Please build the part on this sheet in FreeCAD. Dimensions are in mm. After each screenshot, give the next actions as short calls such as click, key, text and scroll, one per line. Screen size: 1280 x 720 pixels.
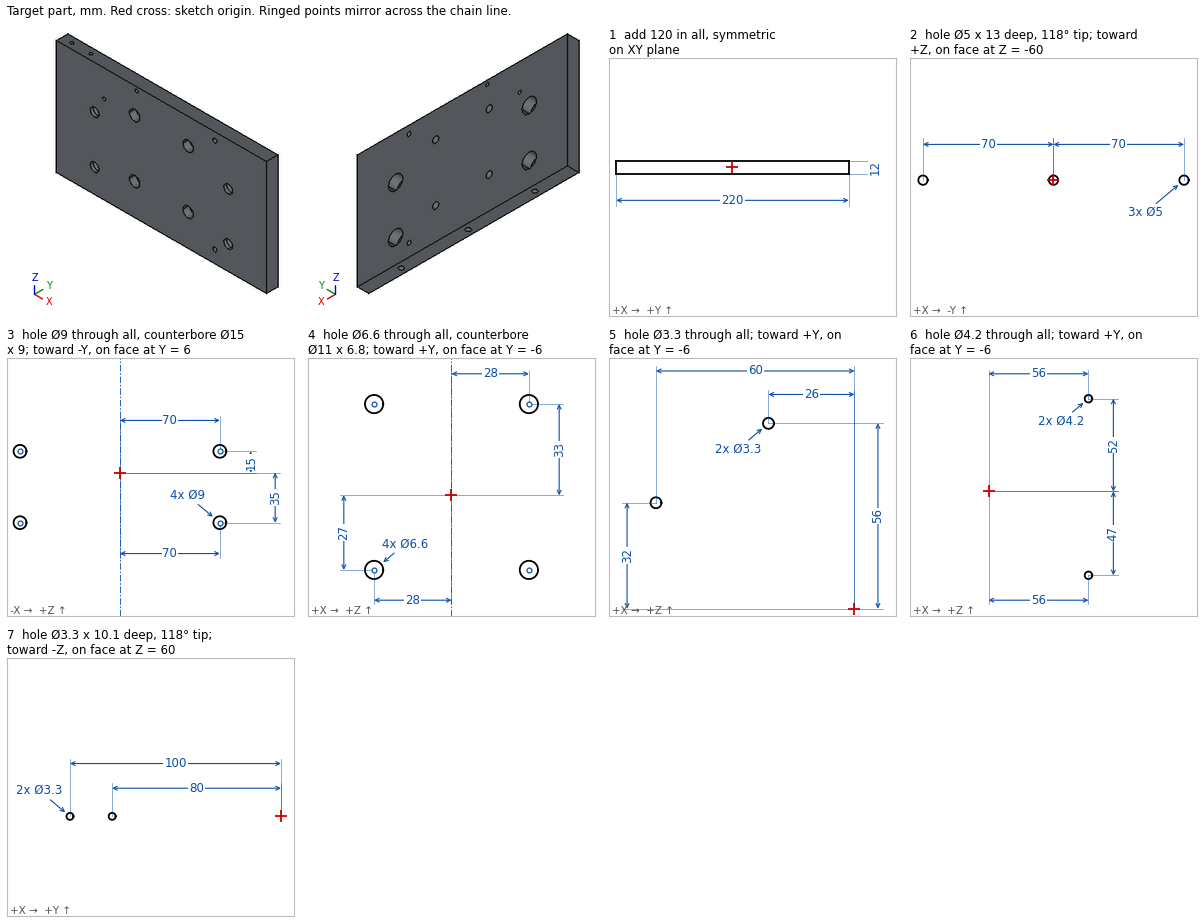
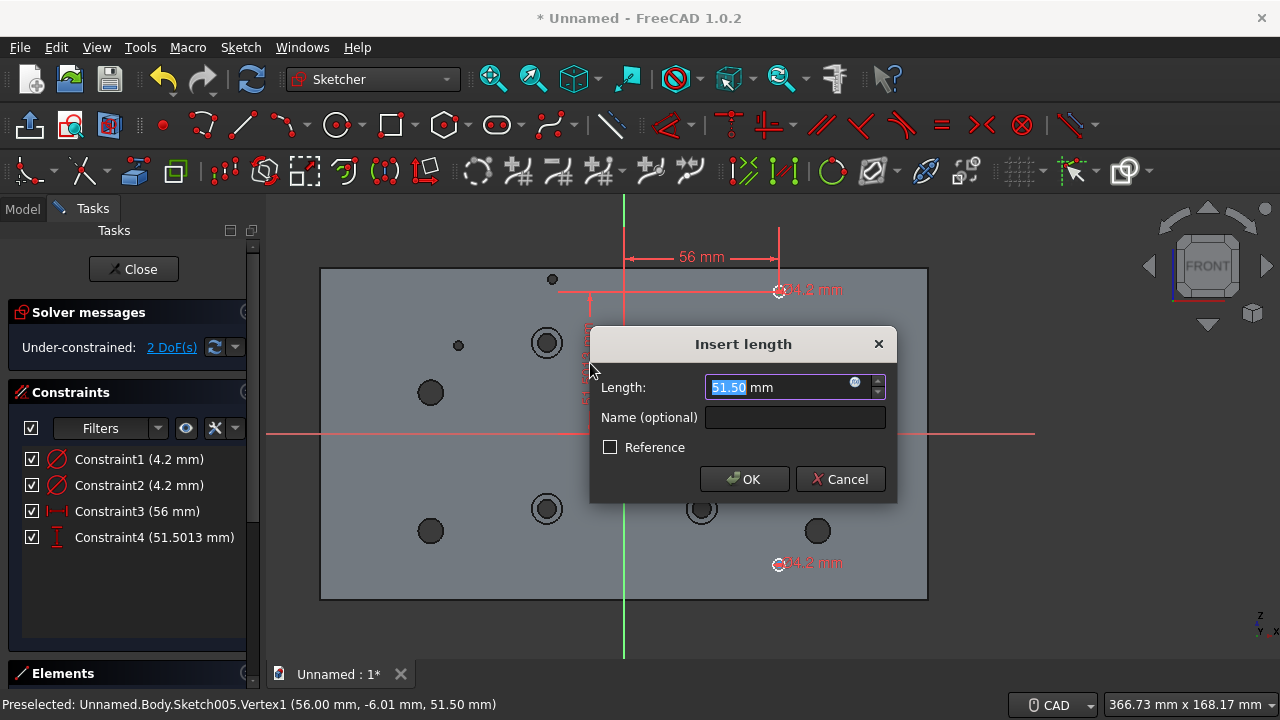
text(52)
key(Return)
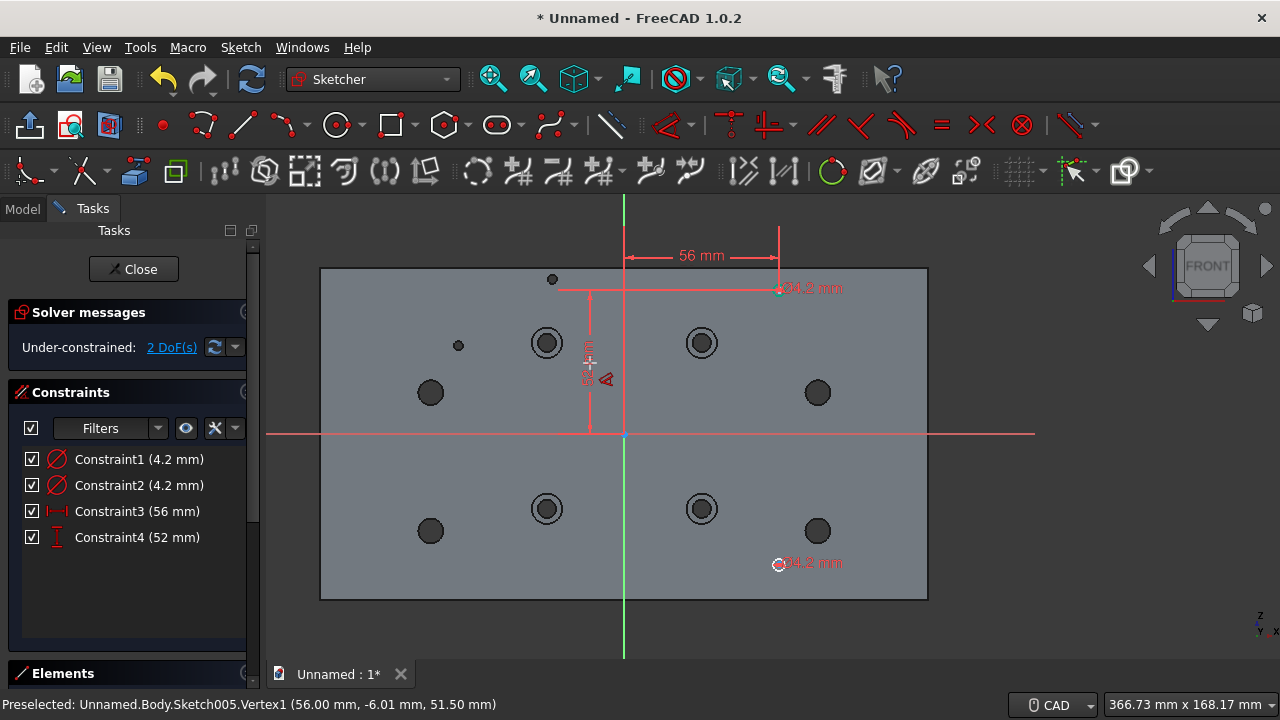
click(779, 565)
click(702, 599)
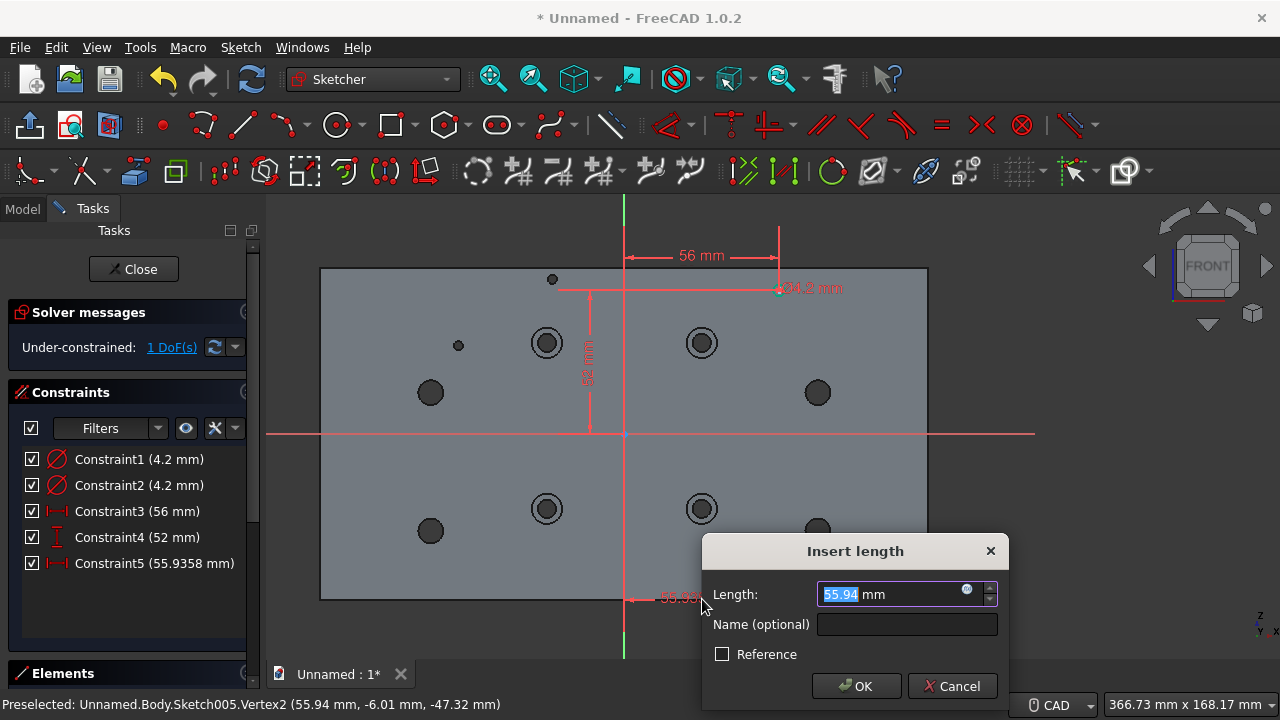
text(56)
key(Return)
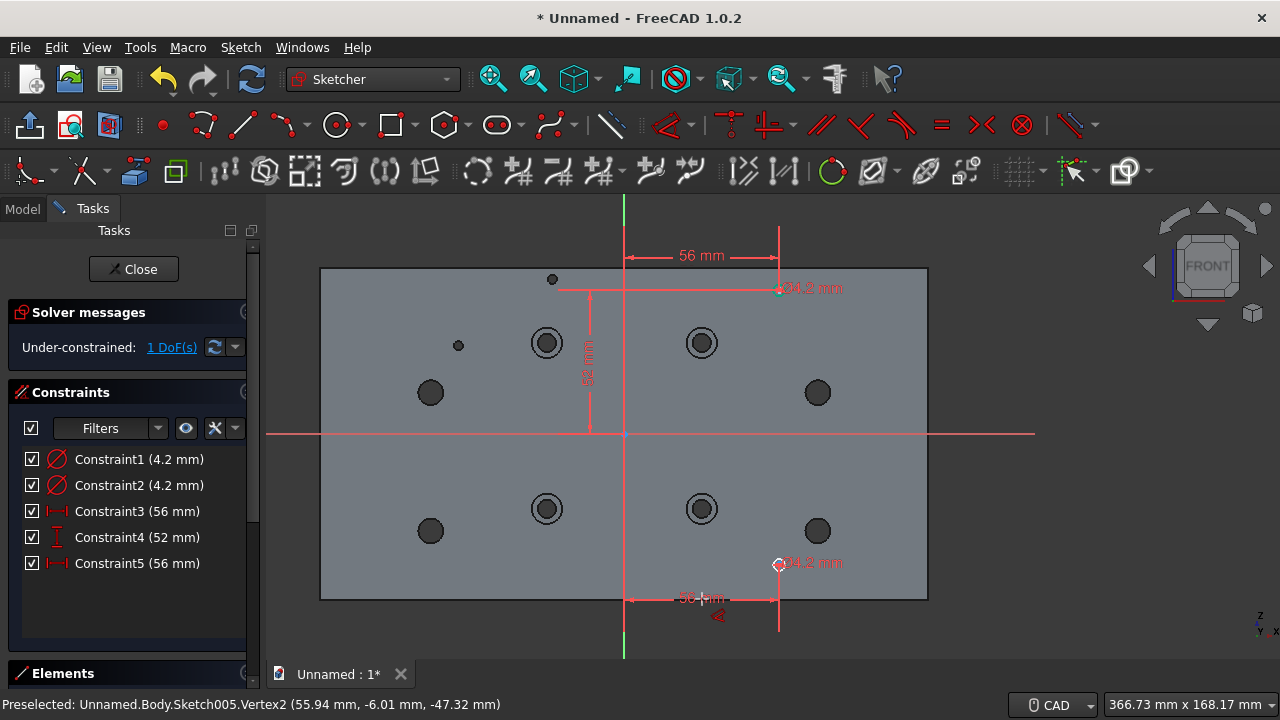
click(779, 565)
click(590, 500)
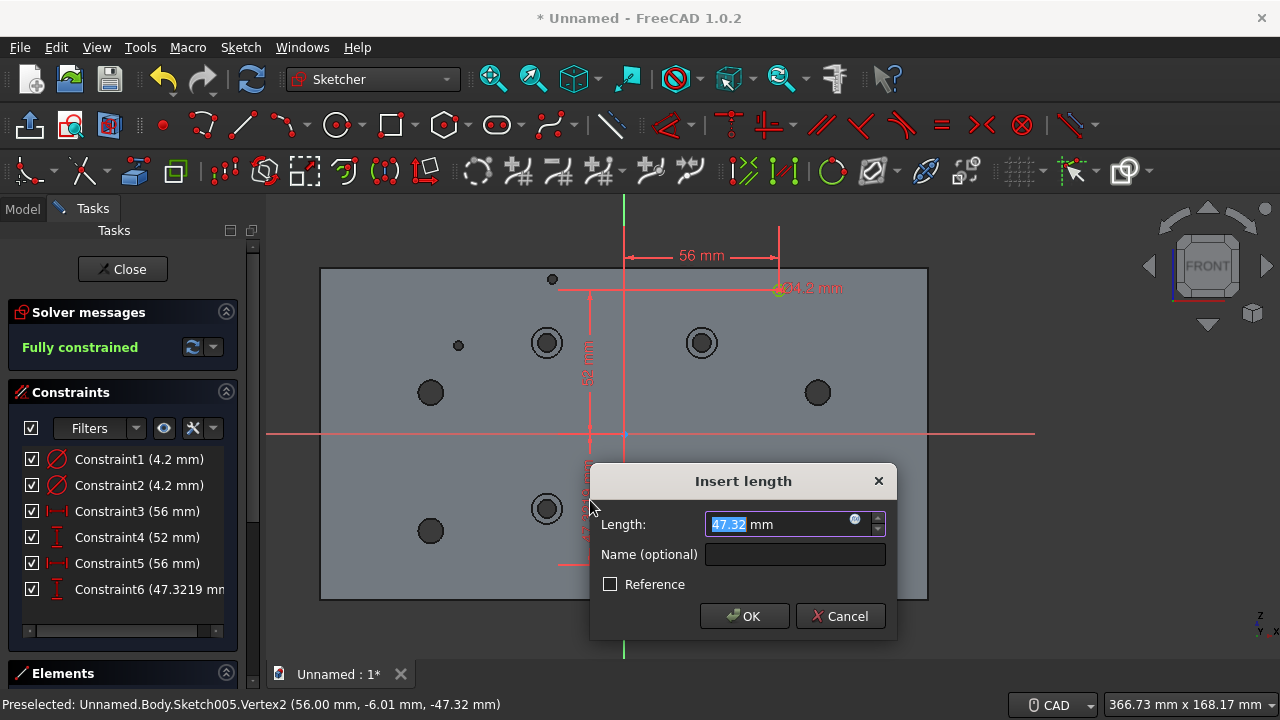
text(47)
key(Return)
key(Escape)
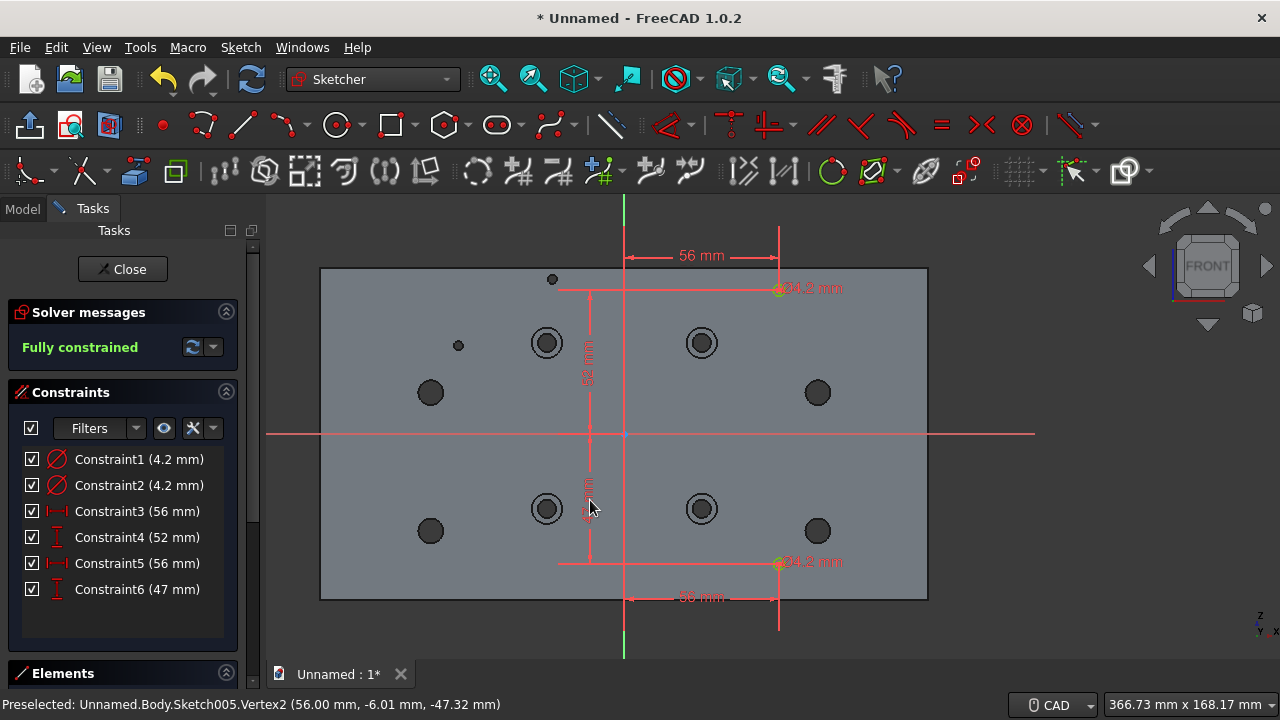
click(123, 269)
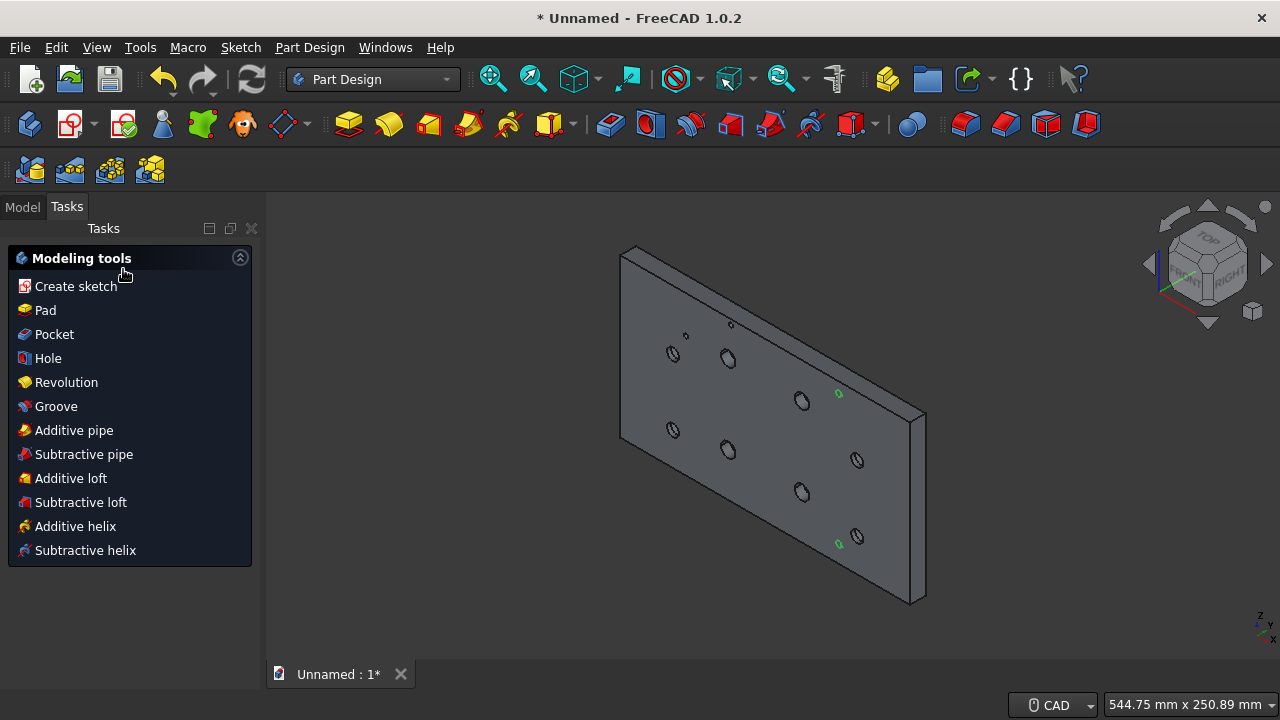
click(652, 124)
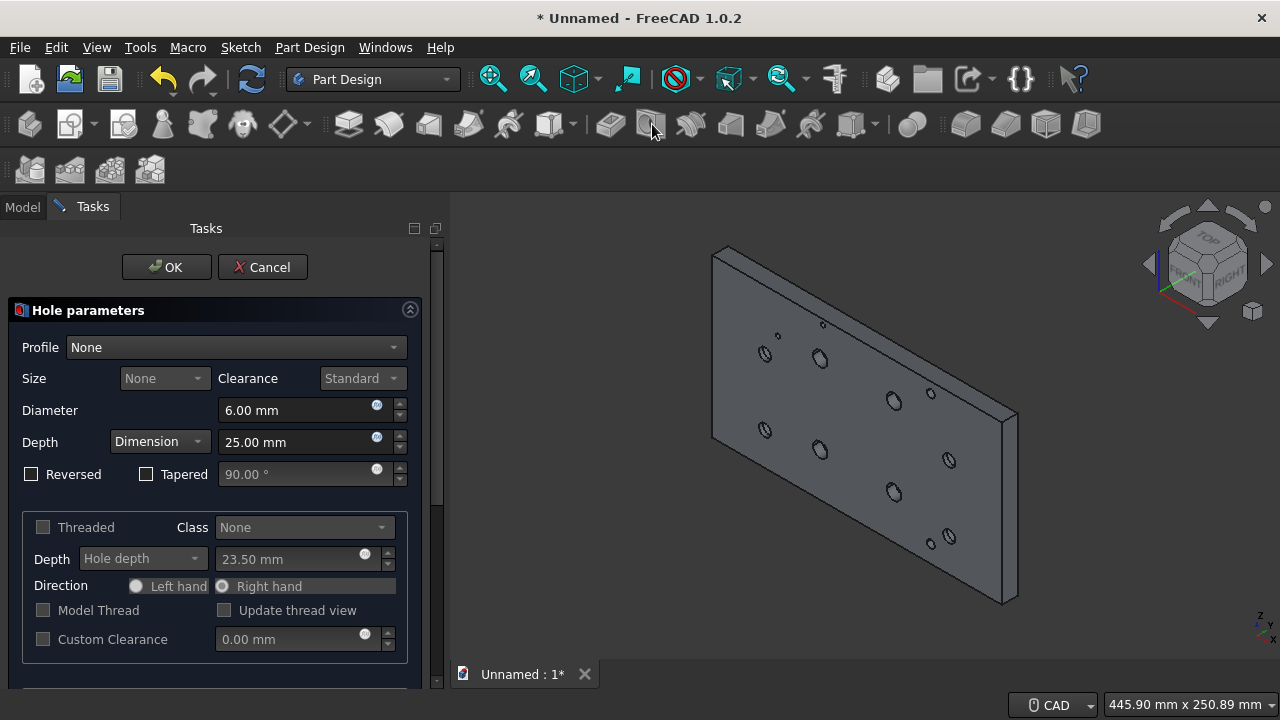
triple_click(305, 410)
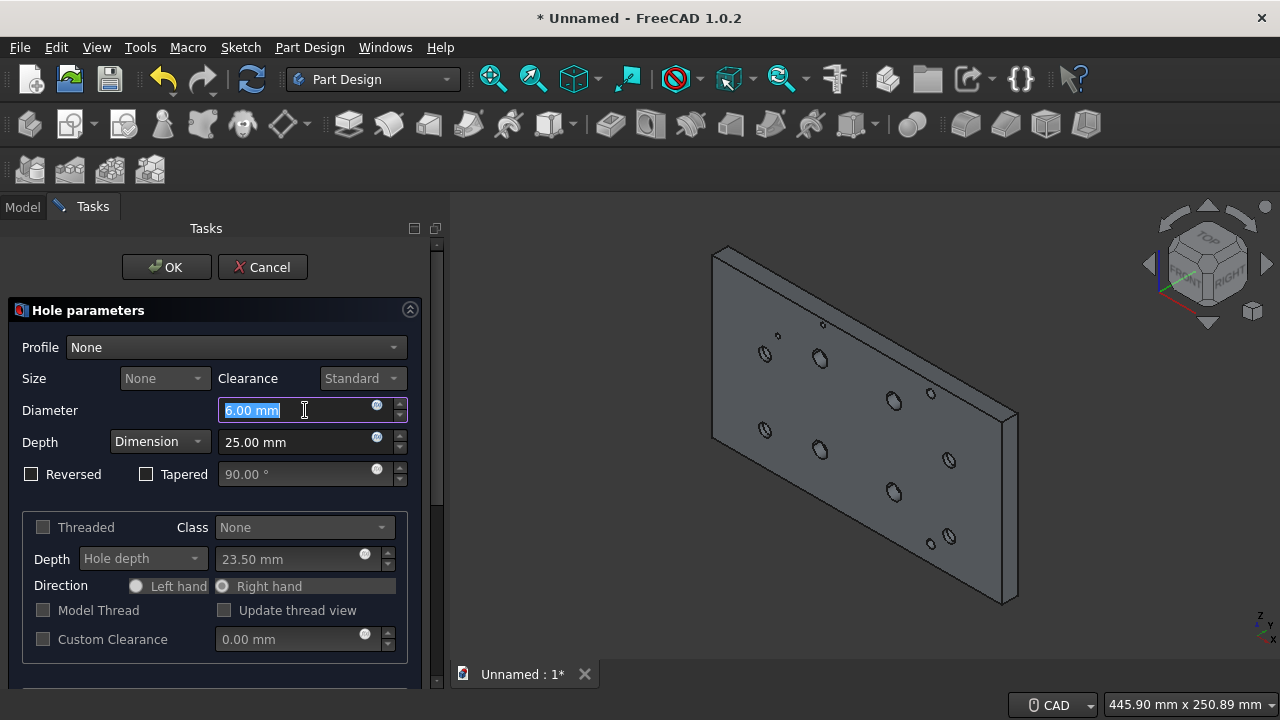
text(4.2)
key(Tab)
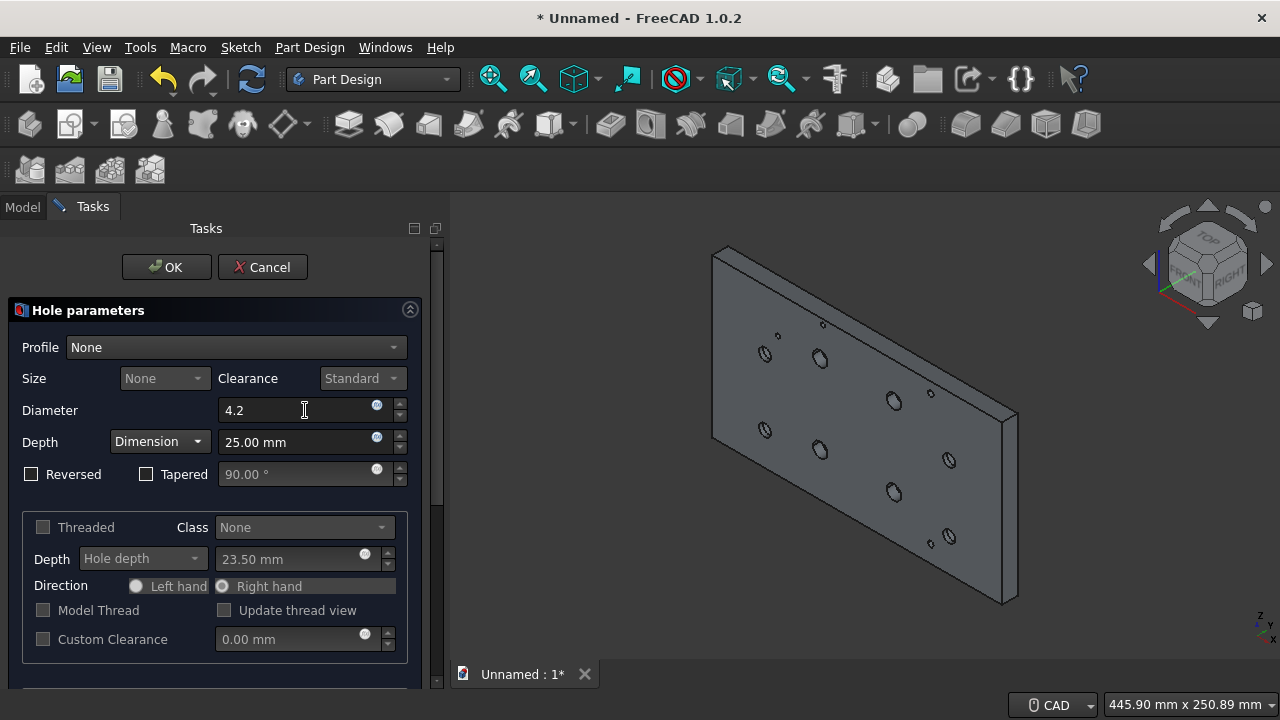
click(161, 442)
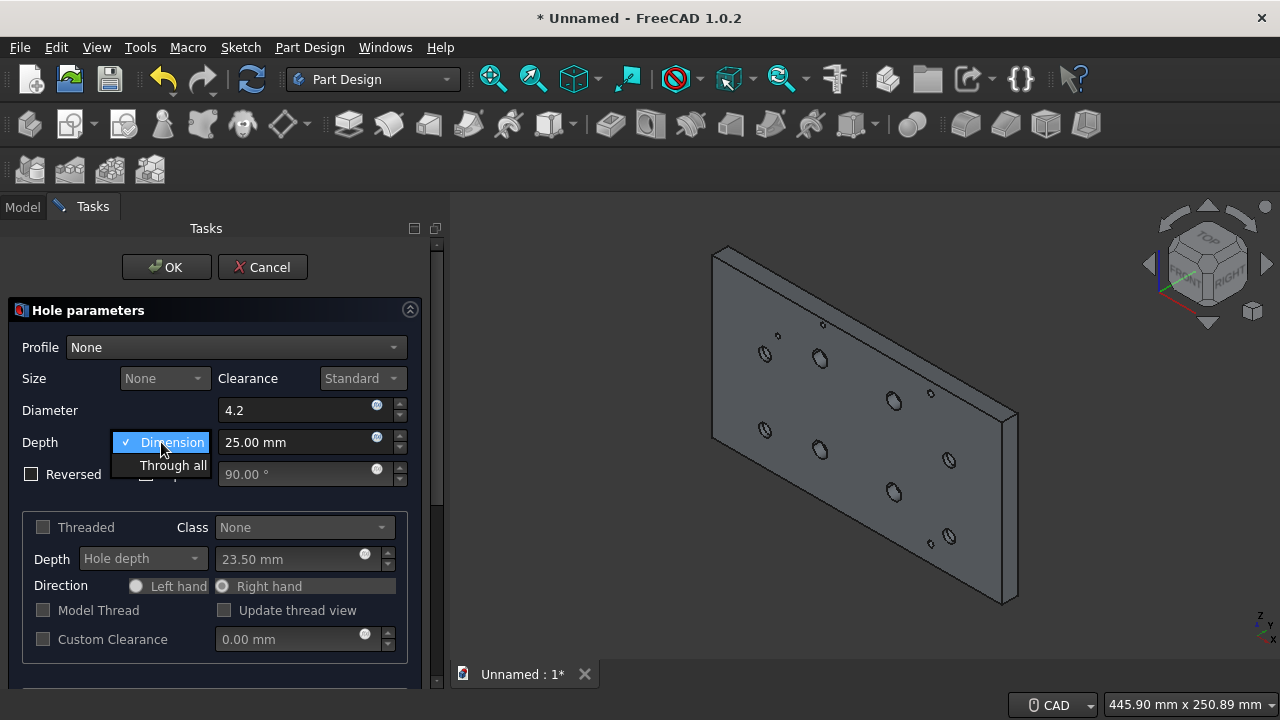
click(160, 466)